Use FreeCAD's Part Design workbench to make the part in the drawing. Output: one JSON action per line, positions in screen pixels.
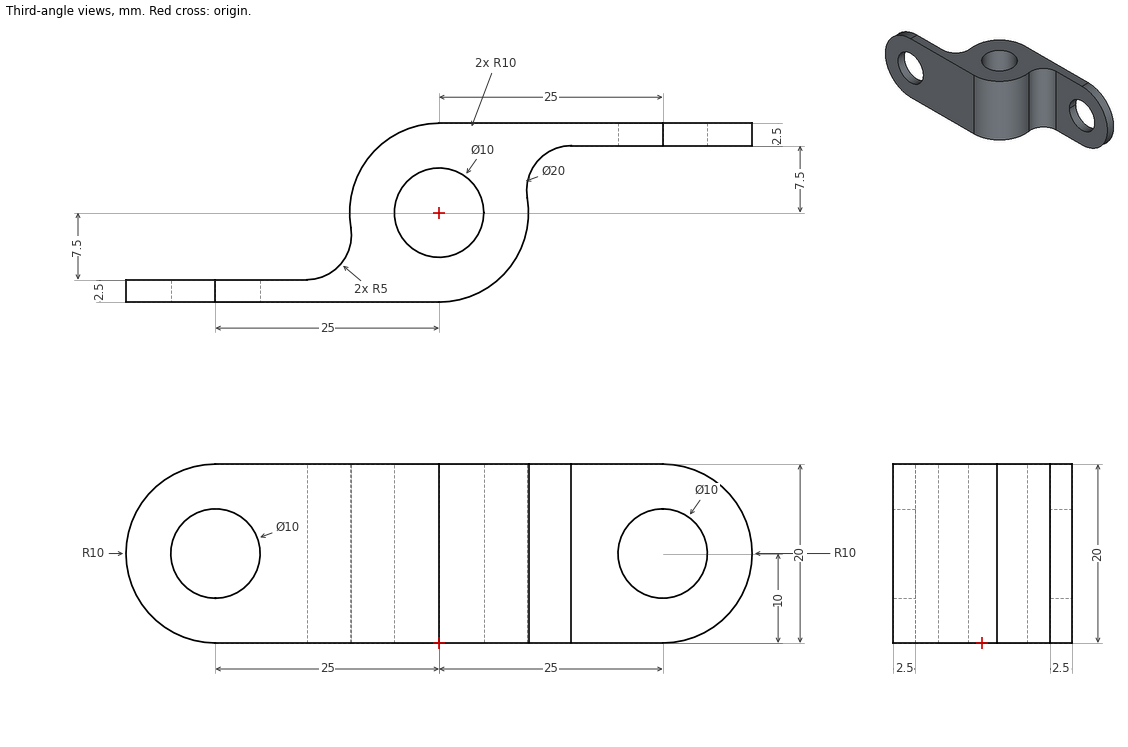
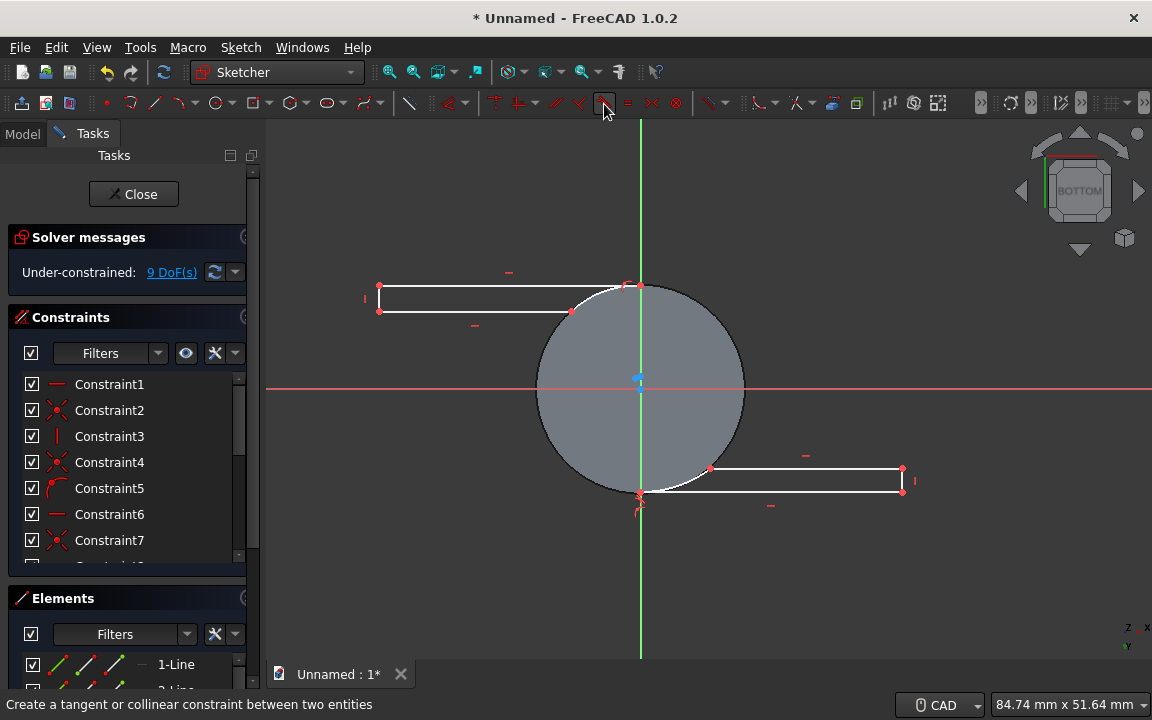
{"action": "left_click", "coordinate": [457, 286]}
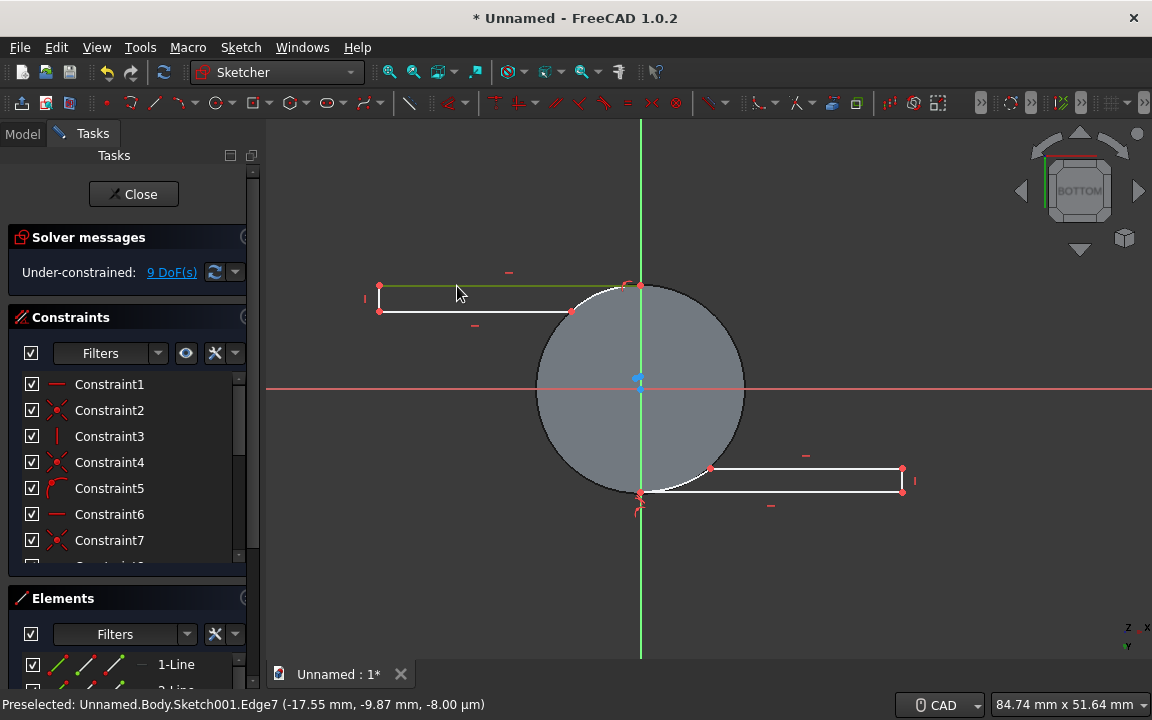
{"action": "left_click", "coordinate": [589, 298]}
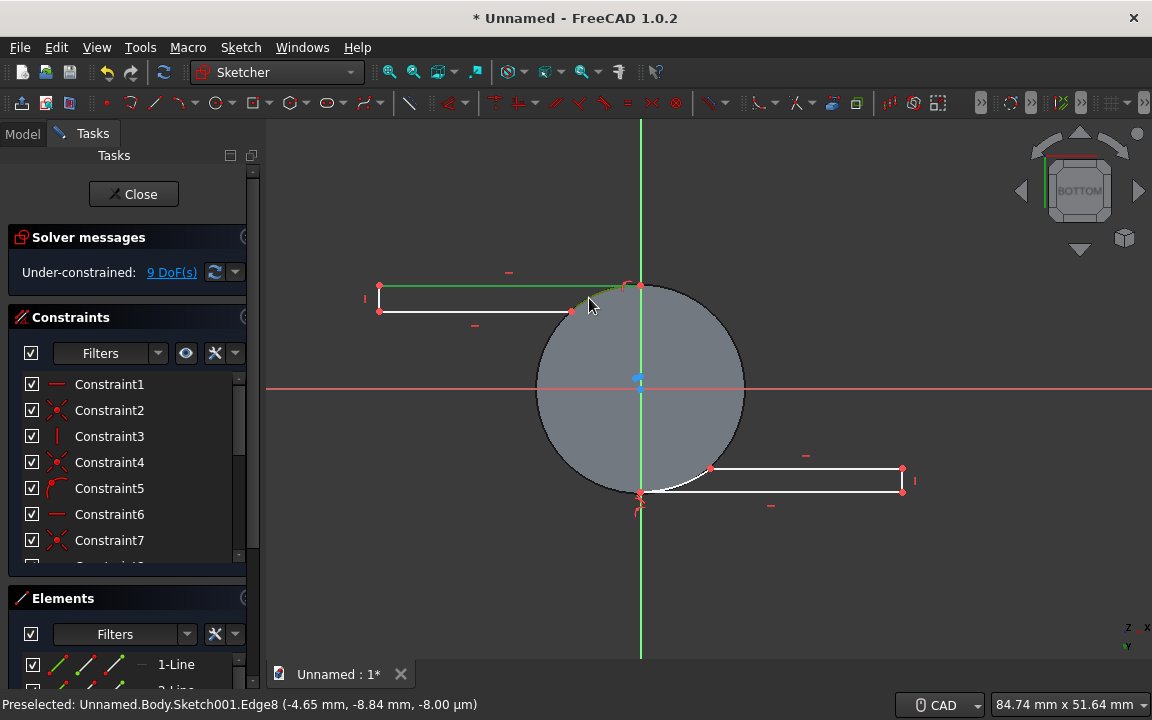
{"action": "left_click", "coordinate": [604, 104]}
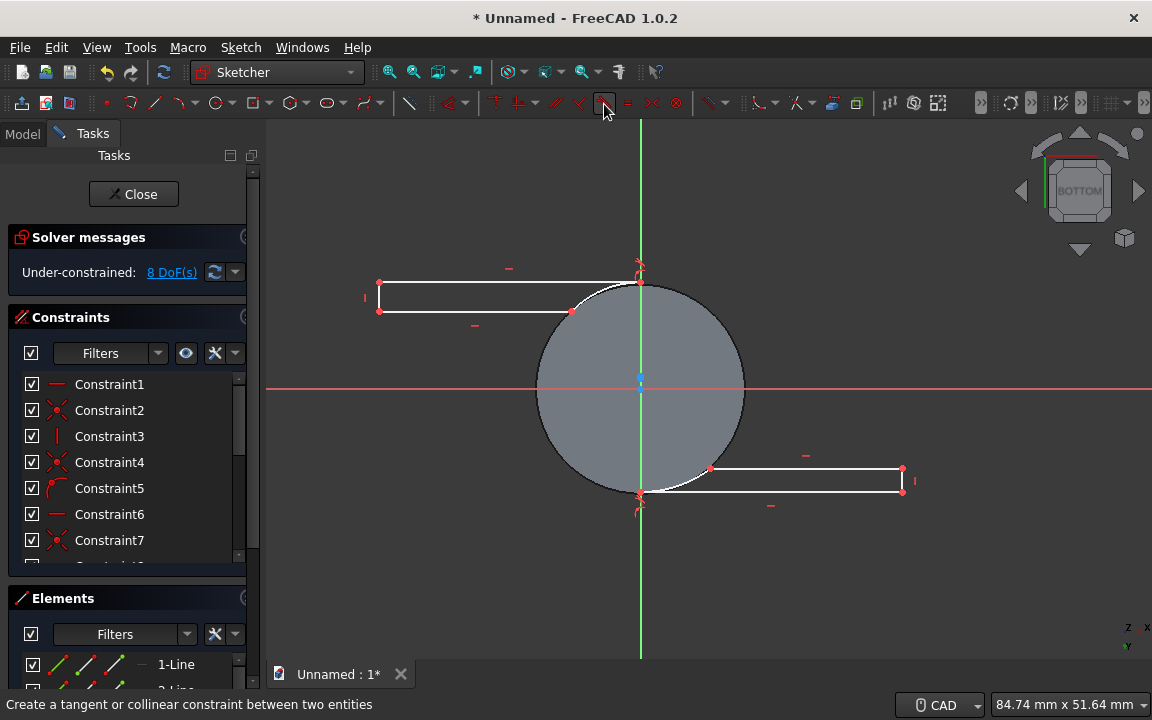
{"action": "left_click", "coordinate": [691, 481]}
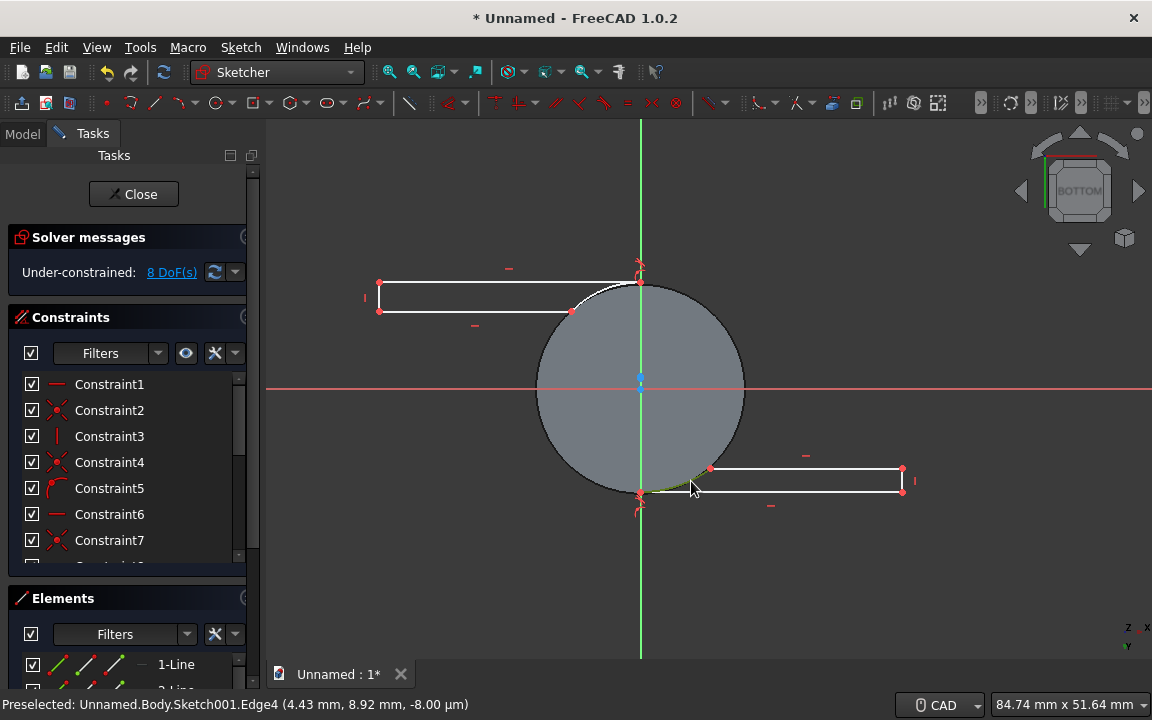
{"action": "left_click", "coordinate": [589, 297]}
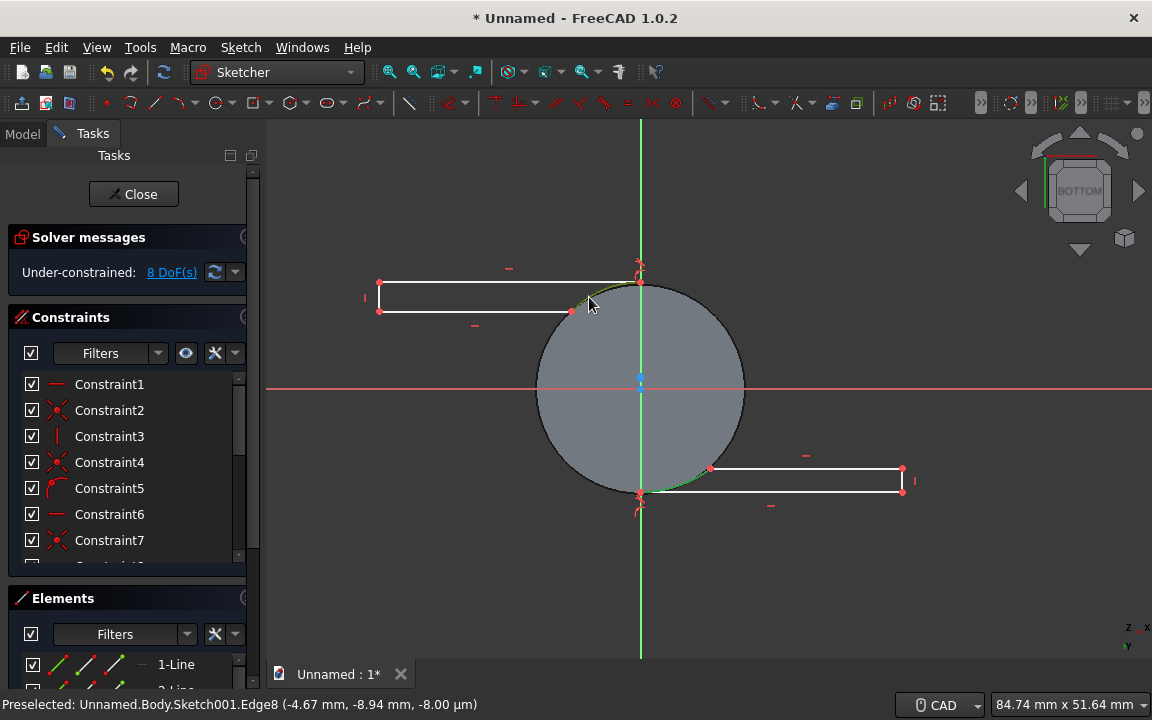
{"action": "key", "text": "e"}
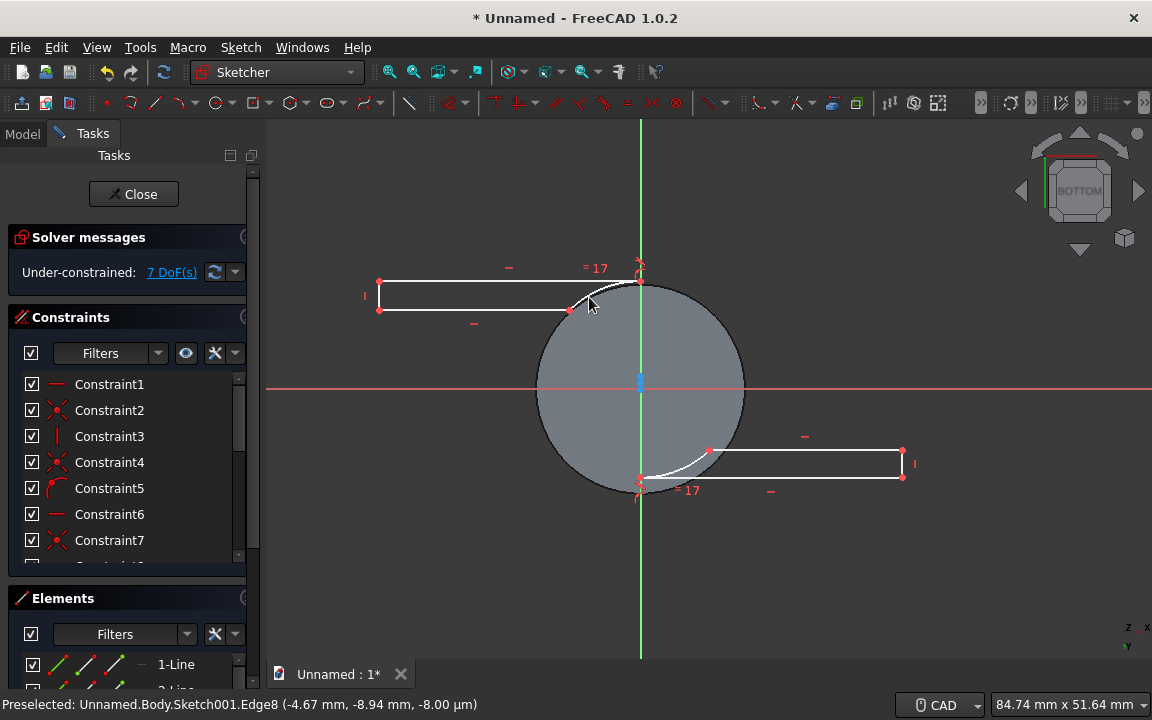
{"action": "left_click", "coordinate": [641, 376]}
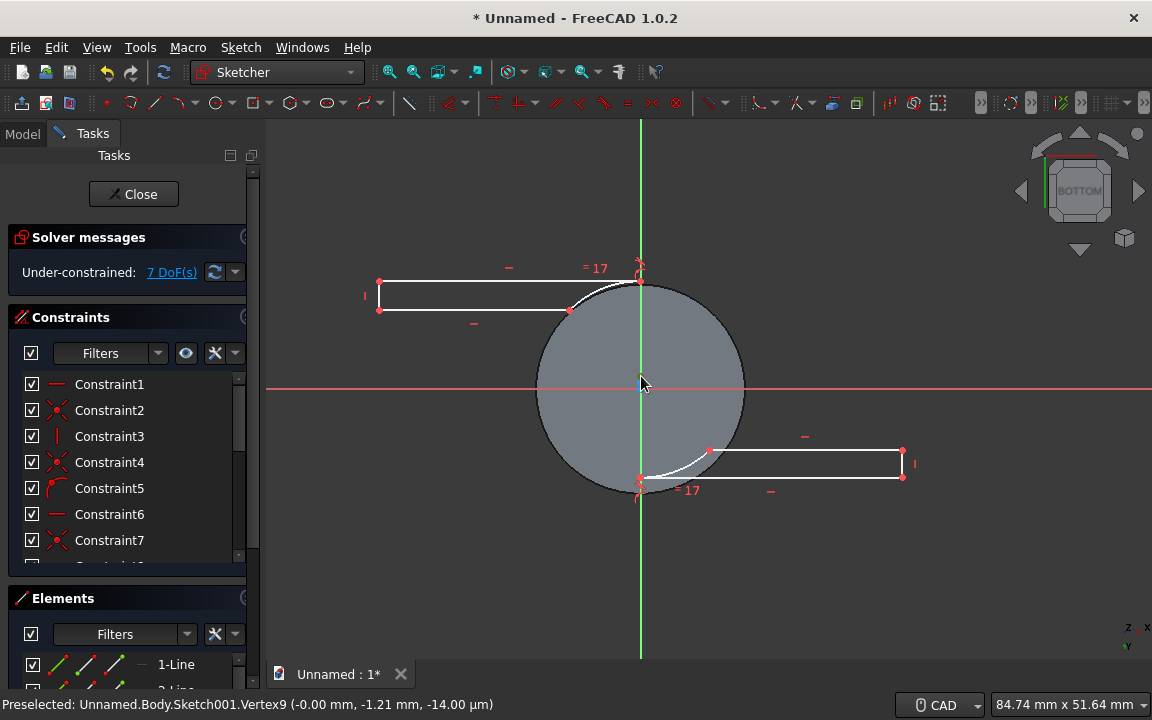
{"action": "left_click", "coordinate": [344, 389]}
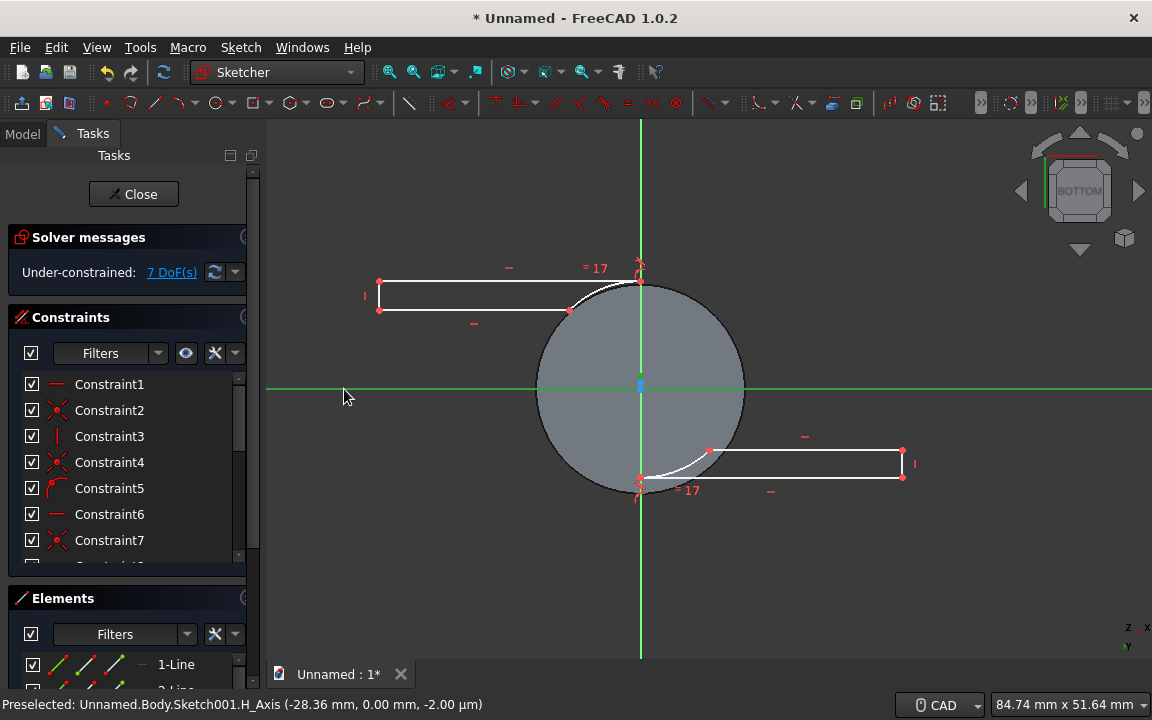
{"action": "left_click", "coordinate": [496, 104]}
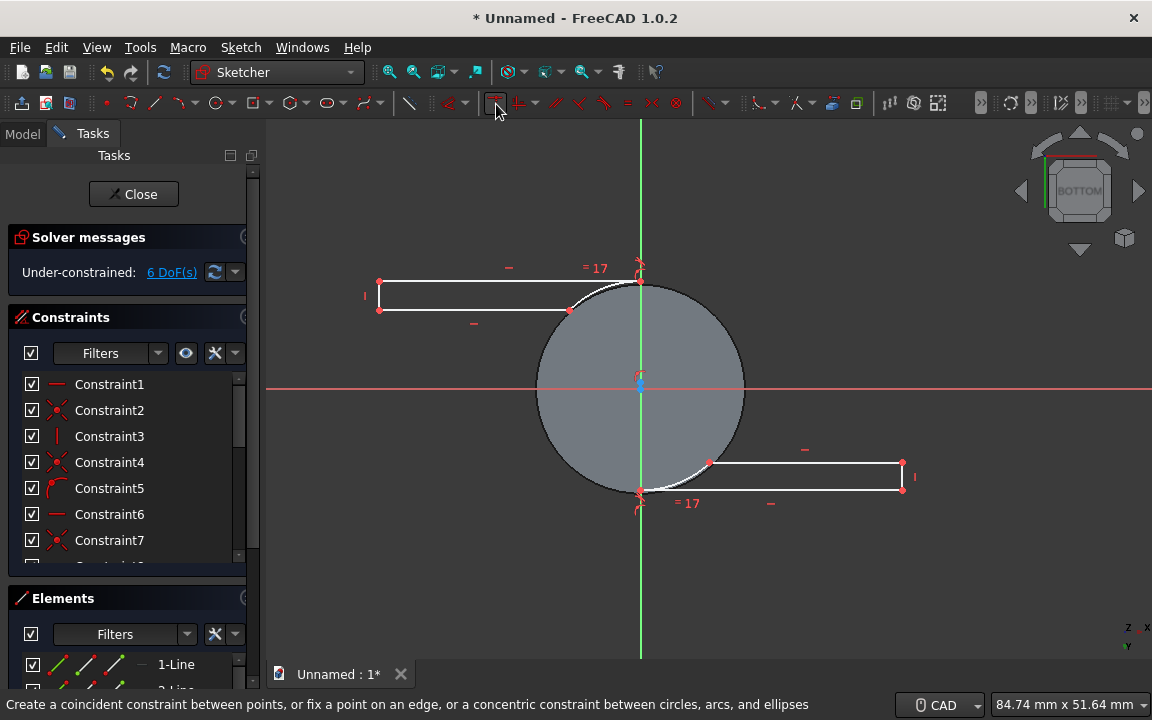
{"action": "left_click", "coordinate": [641, 382]}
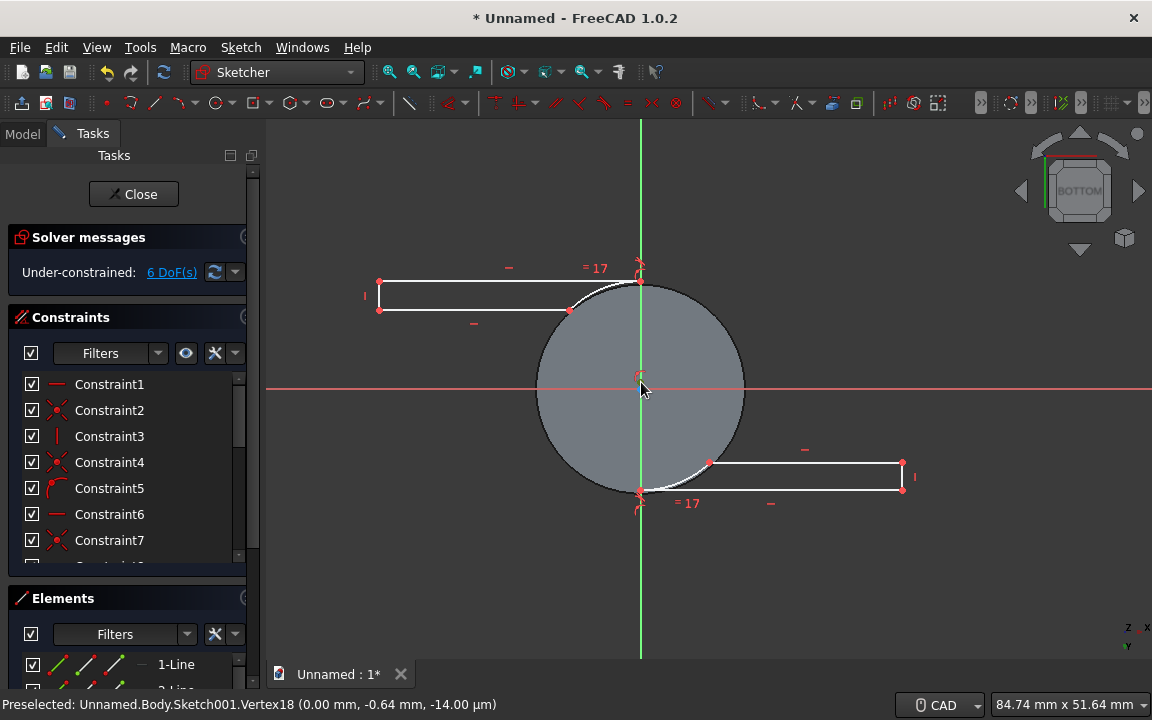
{"action": "left_click", "coordinate": [344, 389]}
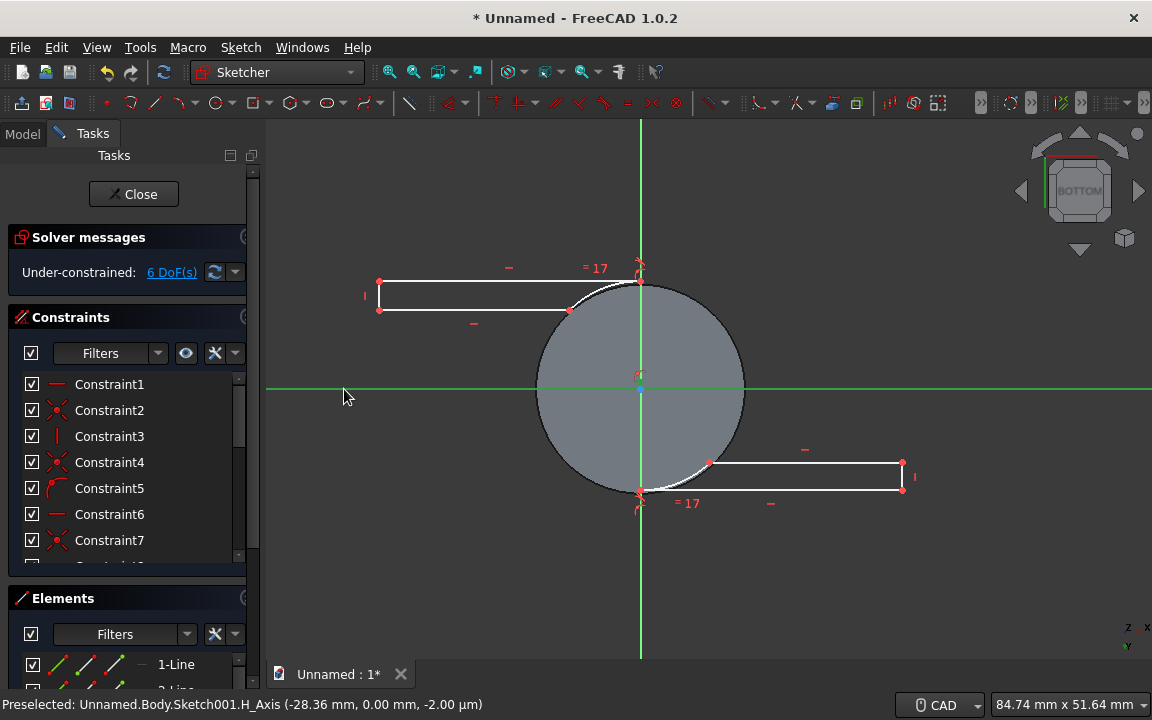
{"action": "key", "text": "c"}